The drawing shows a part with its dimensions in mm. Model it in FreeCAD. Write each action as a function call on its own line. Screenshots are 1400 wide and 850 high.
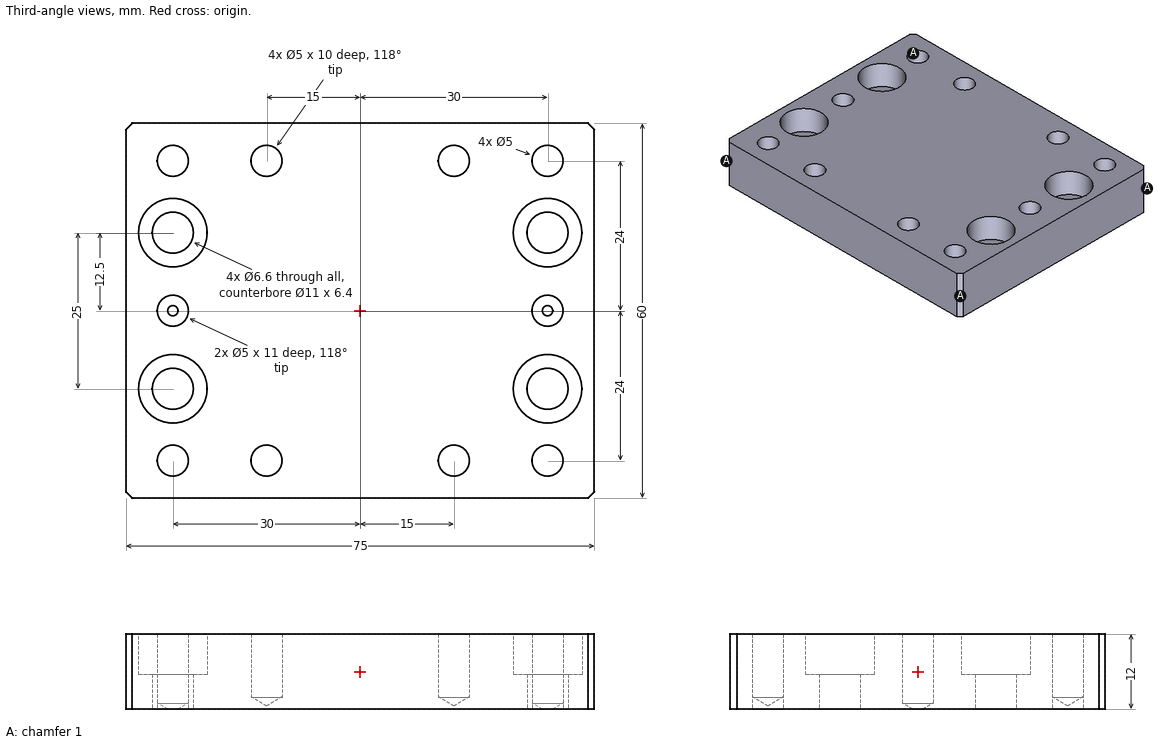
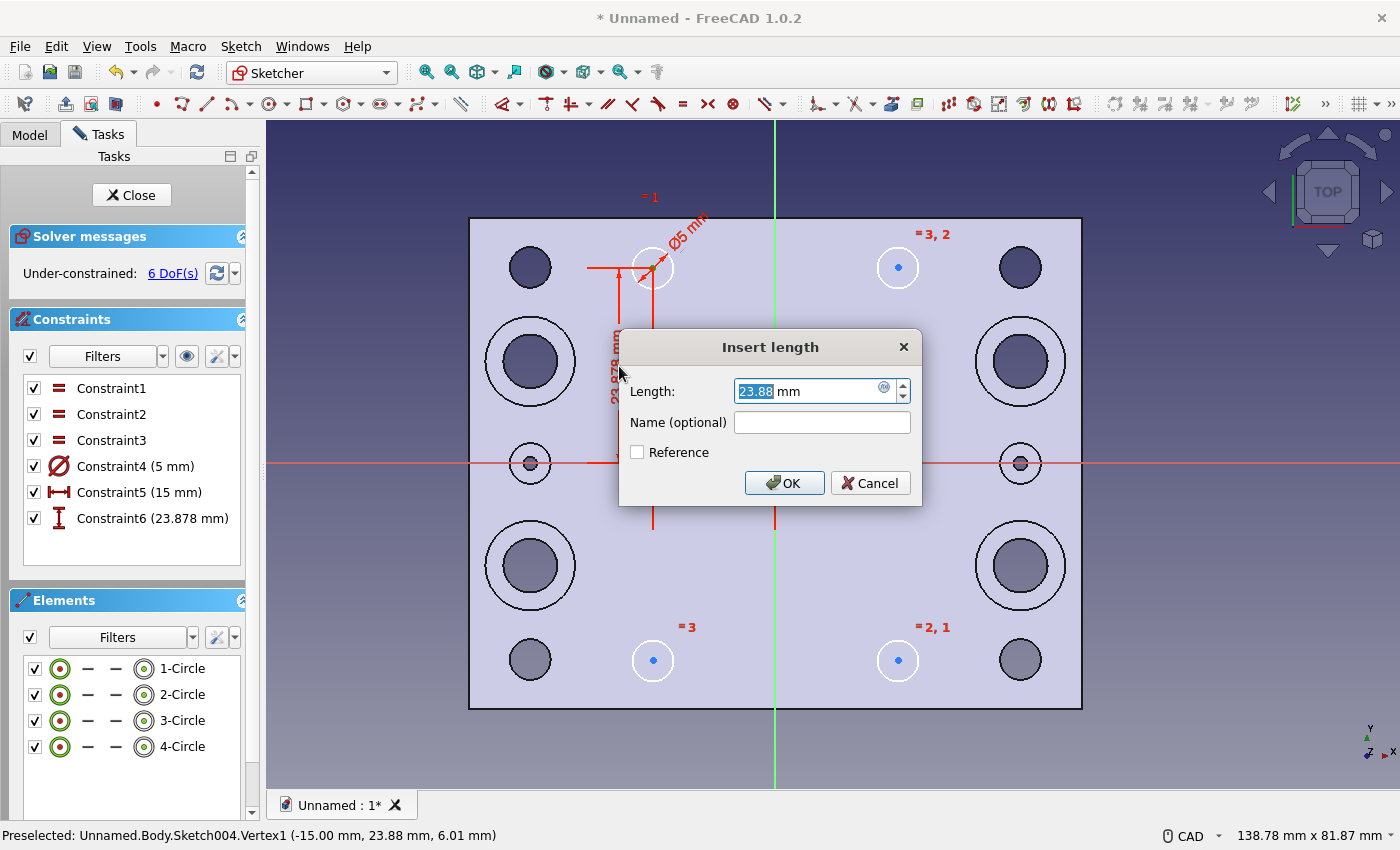
text(24)
key(Return)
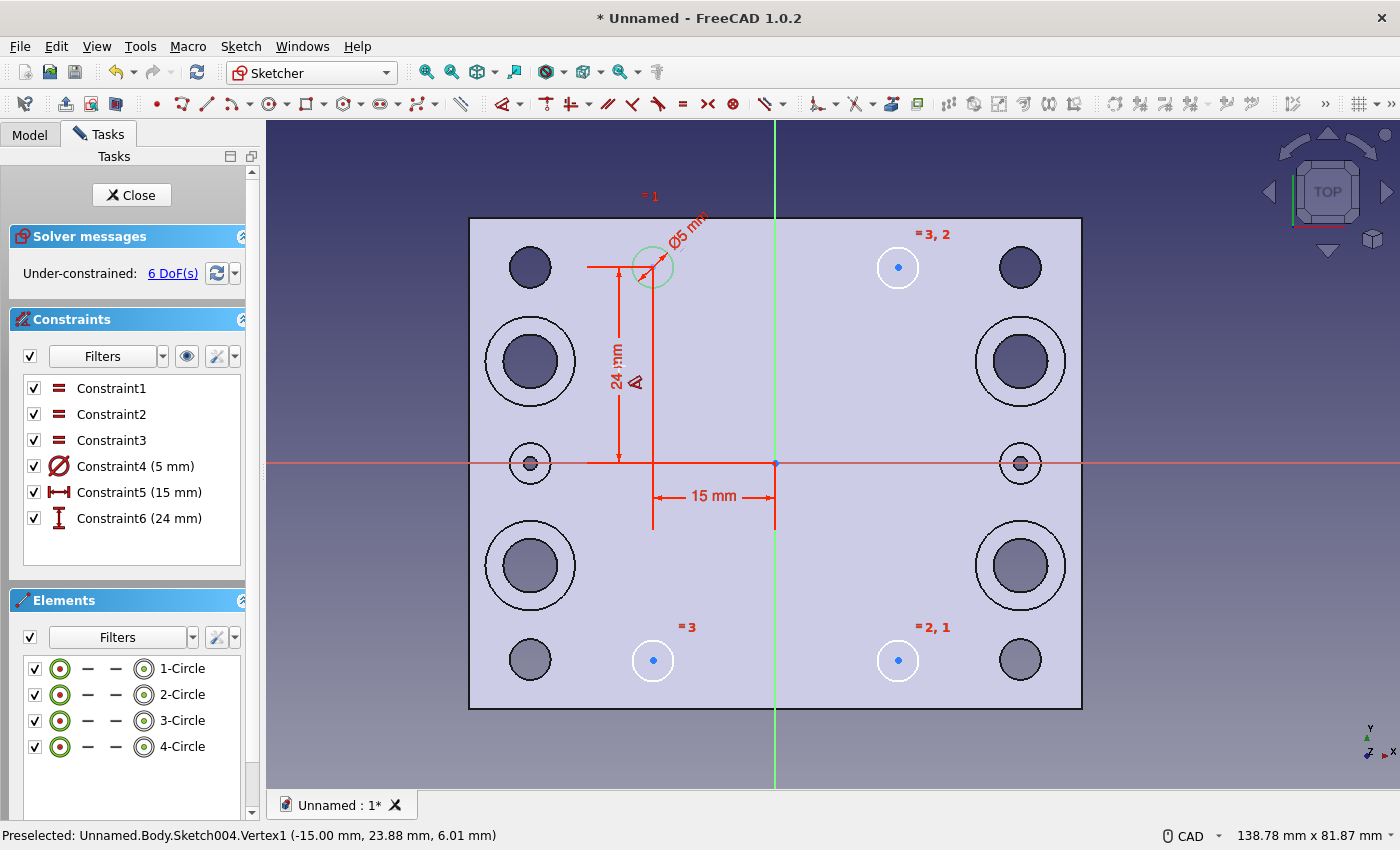
click(898, 661)
click(837, 695)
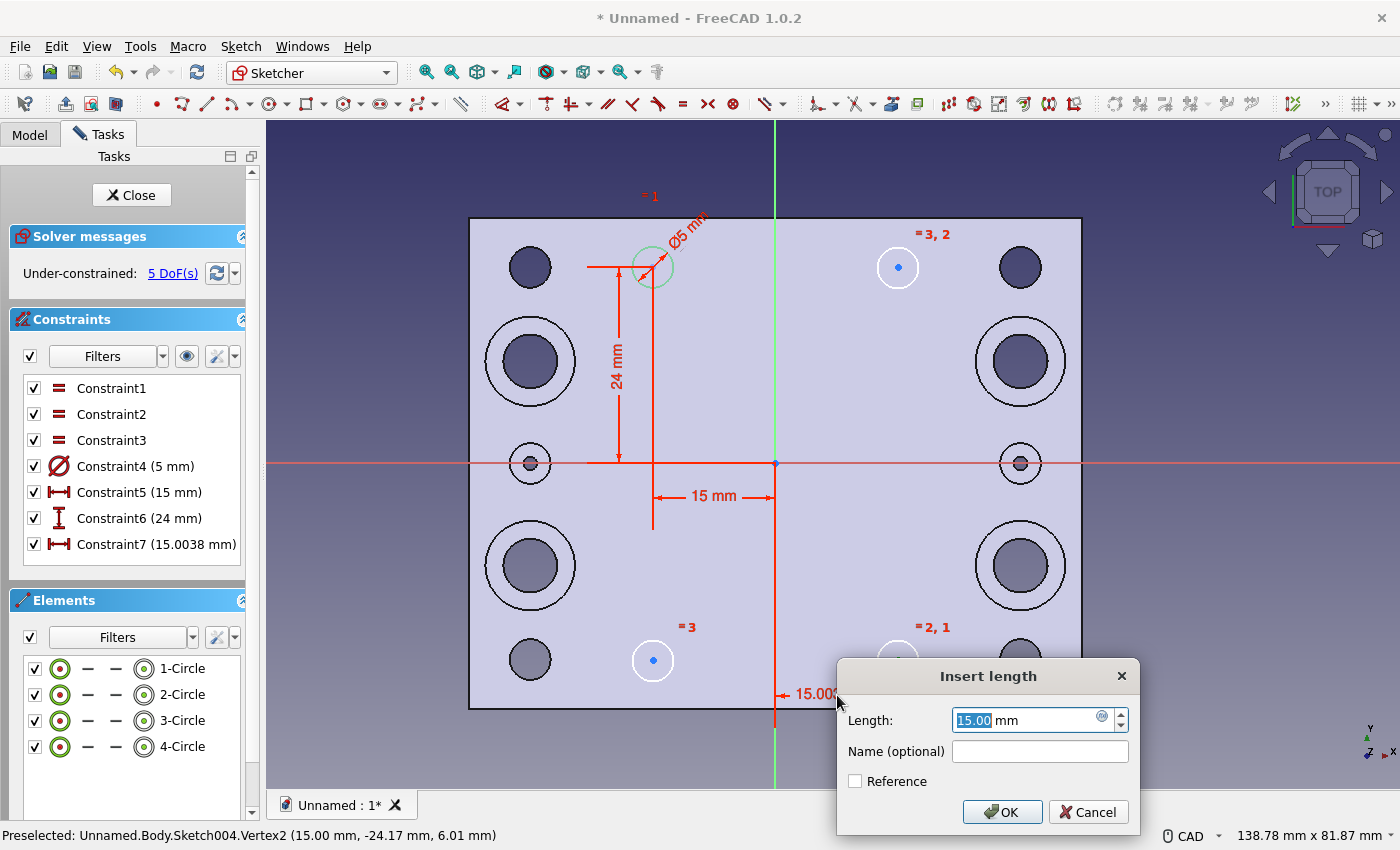
text(15)
key(Return)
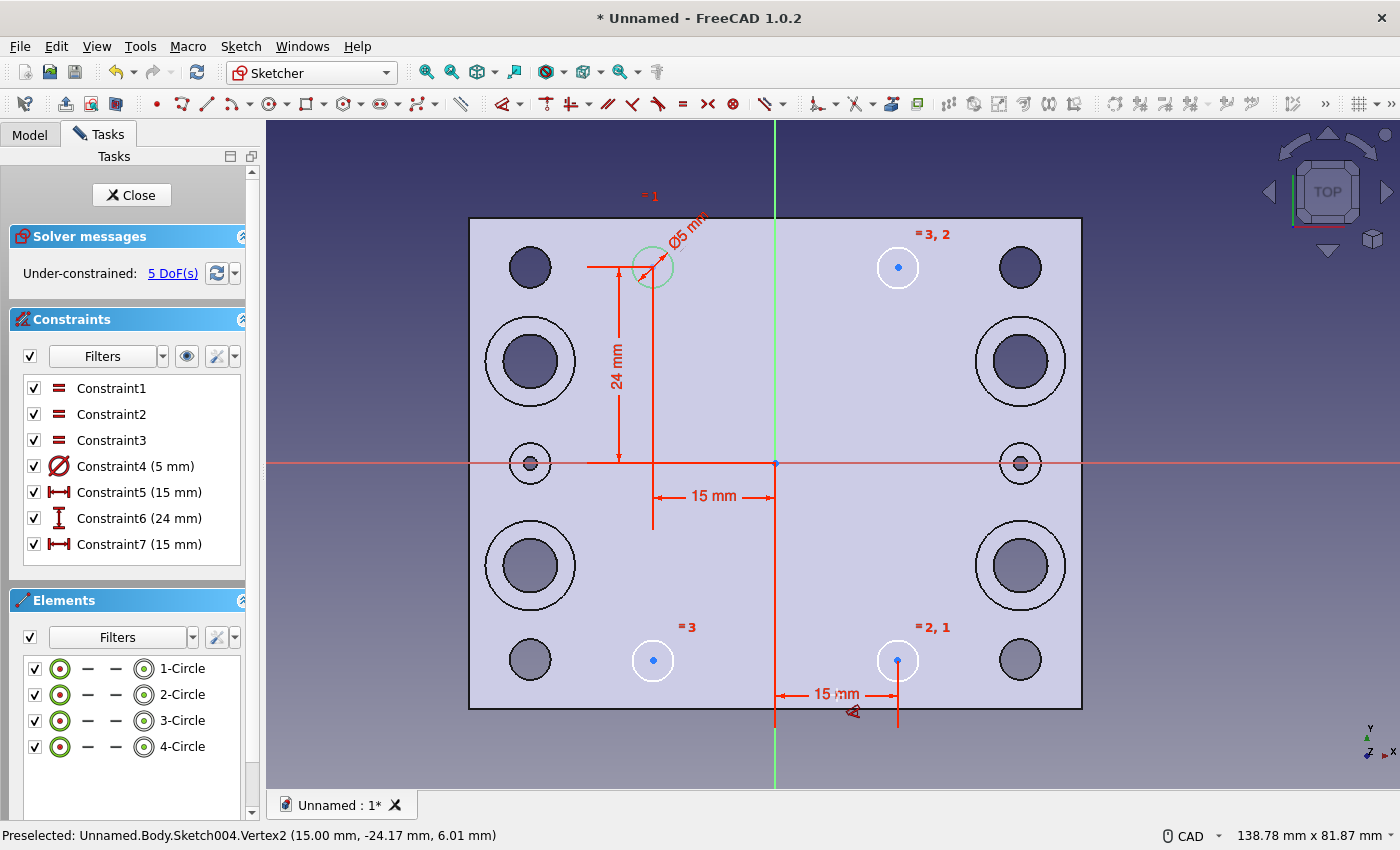
click(898, 661)
click(932, 562)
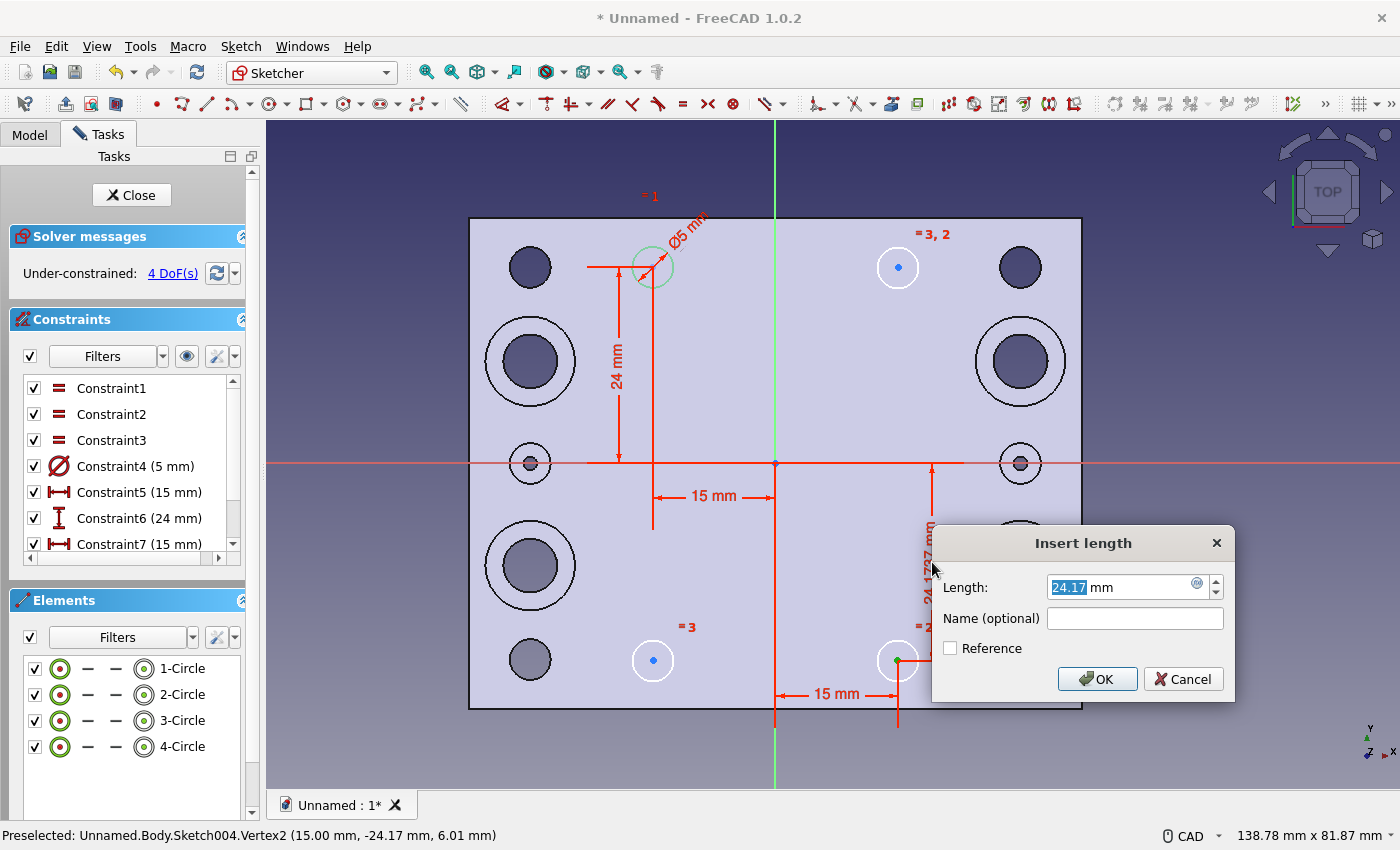
text(24)
key(Return)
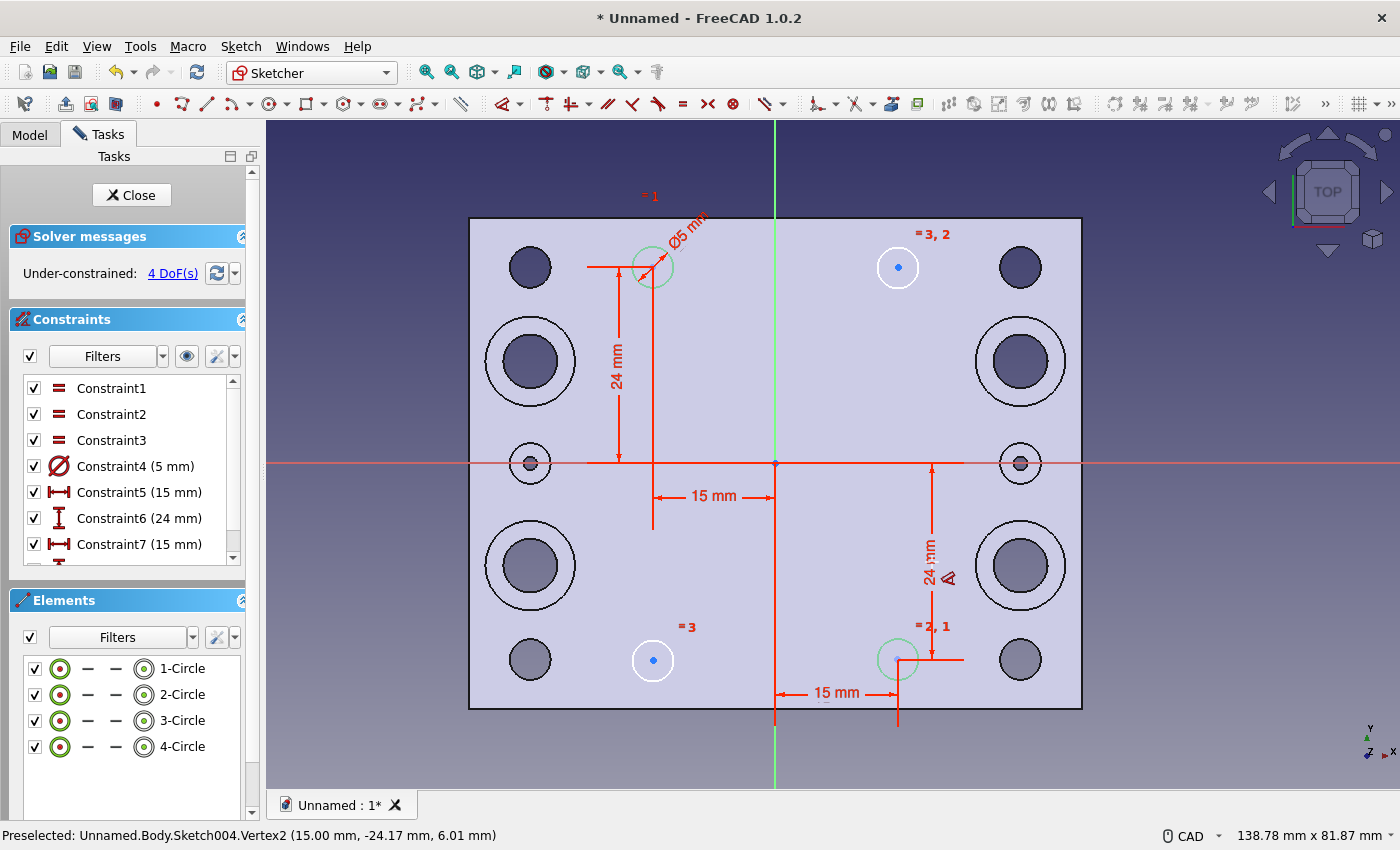
click(898, 268)
click(837, 234)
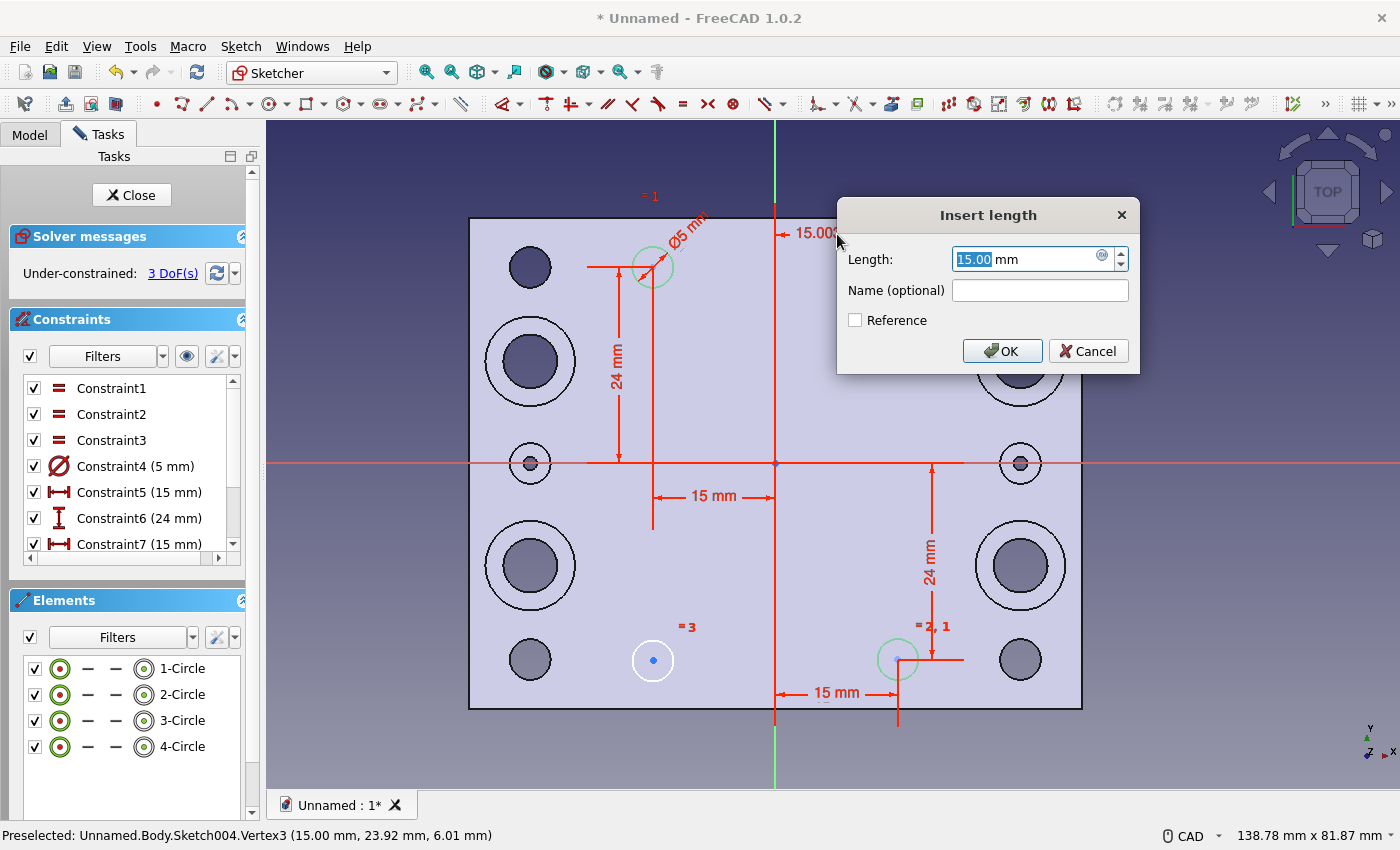
text(15)
key(Return)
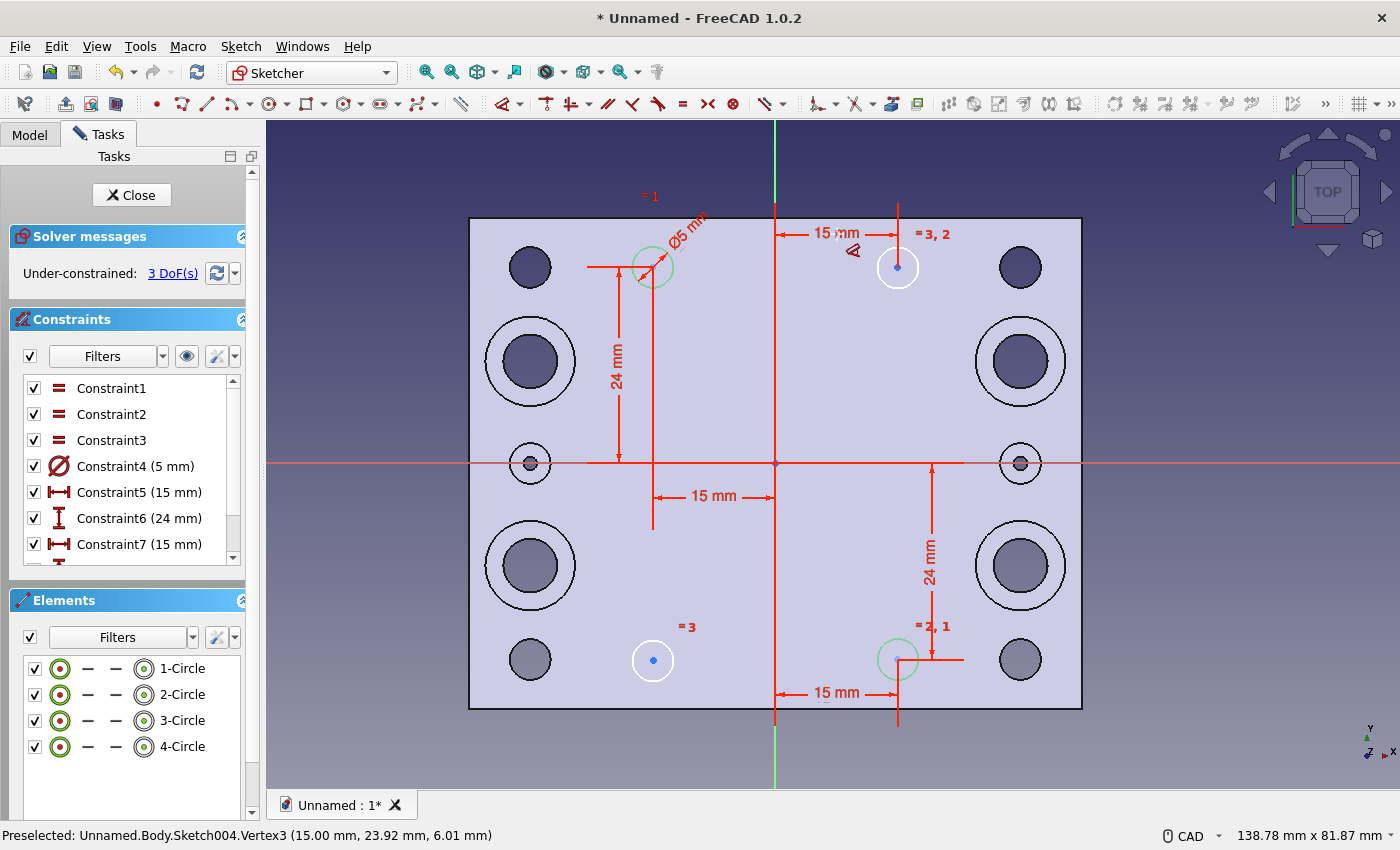
click(898, 268)
click(932, 366)